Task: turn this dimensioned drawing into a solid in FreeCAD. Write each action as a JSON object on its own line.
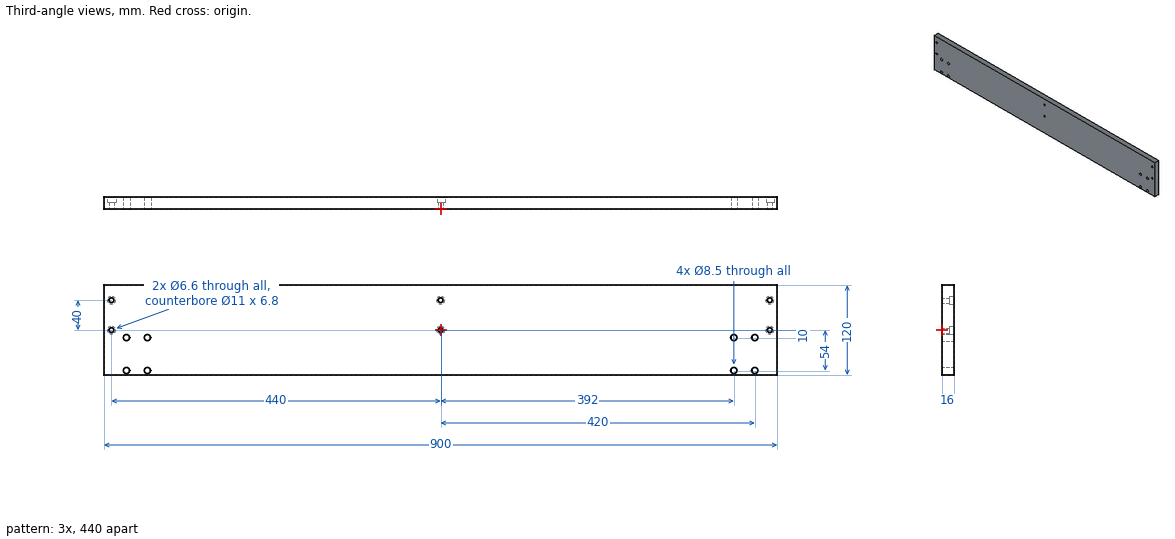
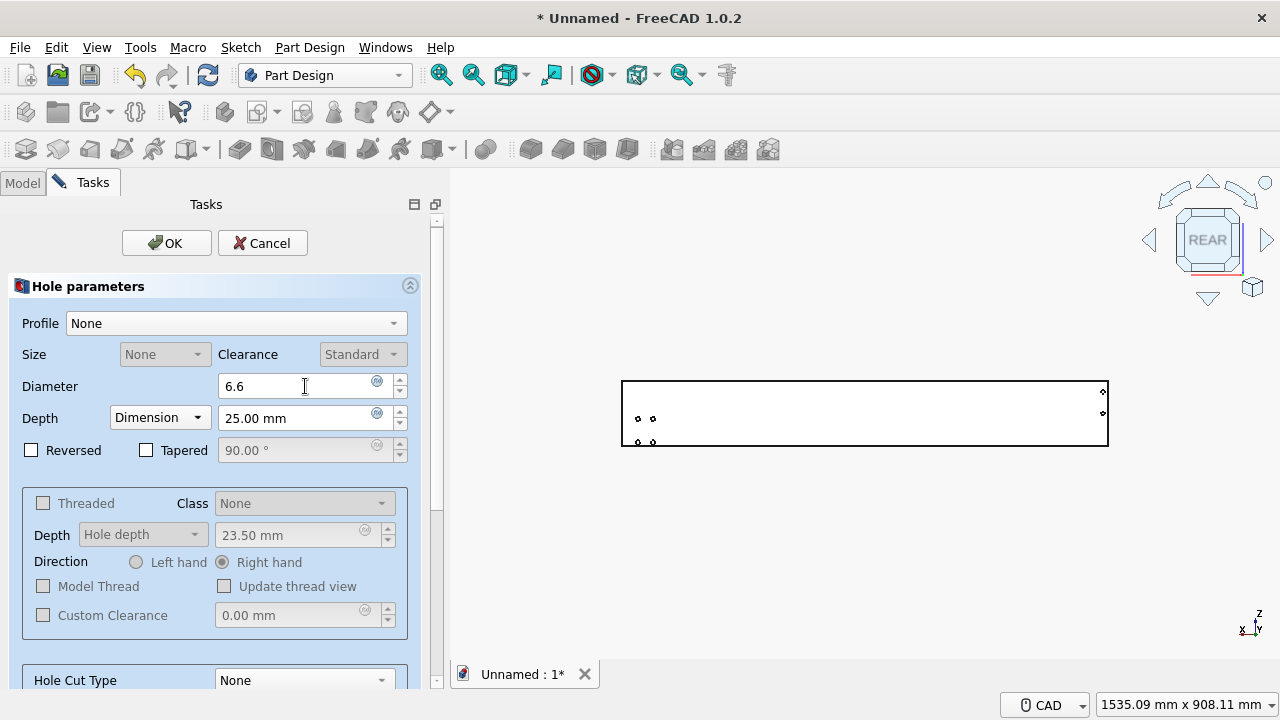
{"action": "left_click", "coordinate": [161, 418]}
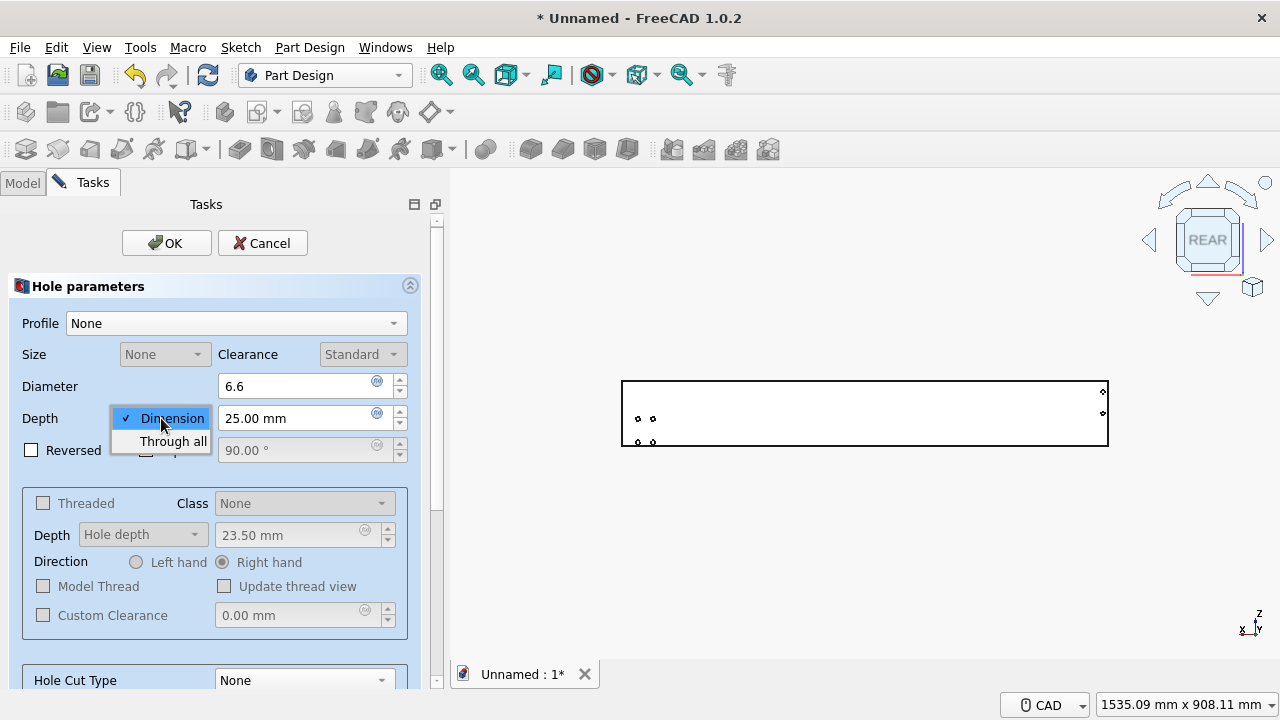
{"action": "left_click", "coordinate": [160, 442]}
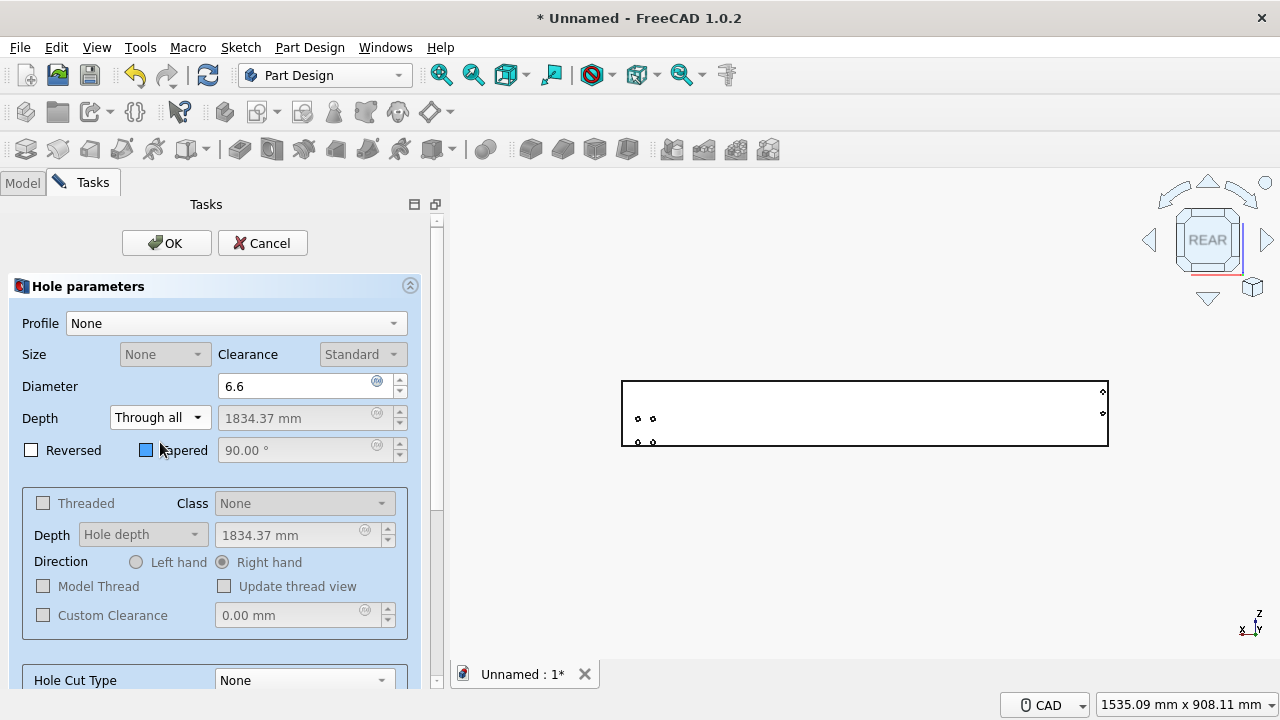
{"action": "scroll", "coordinate": [437, 451], "scroll_direction": "down", "scroll_amount": 2}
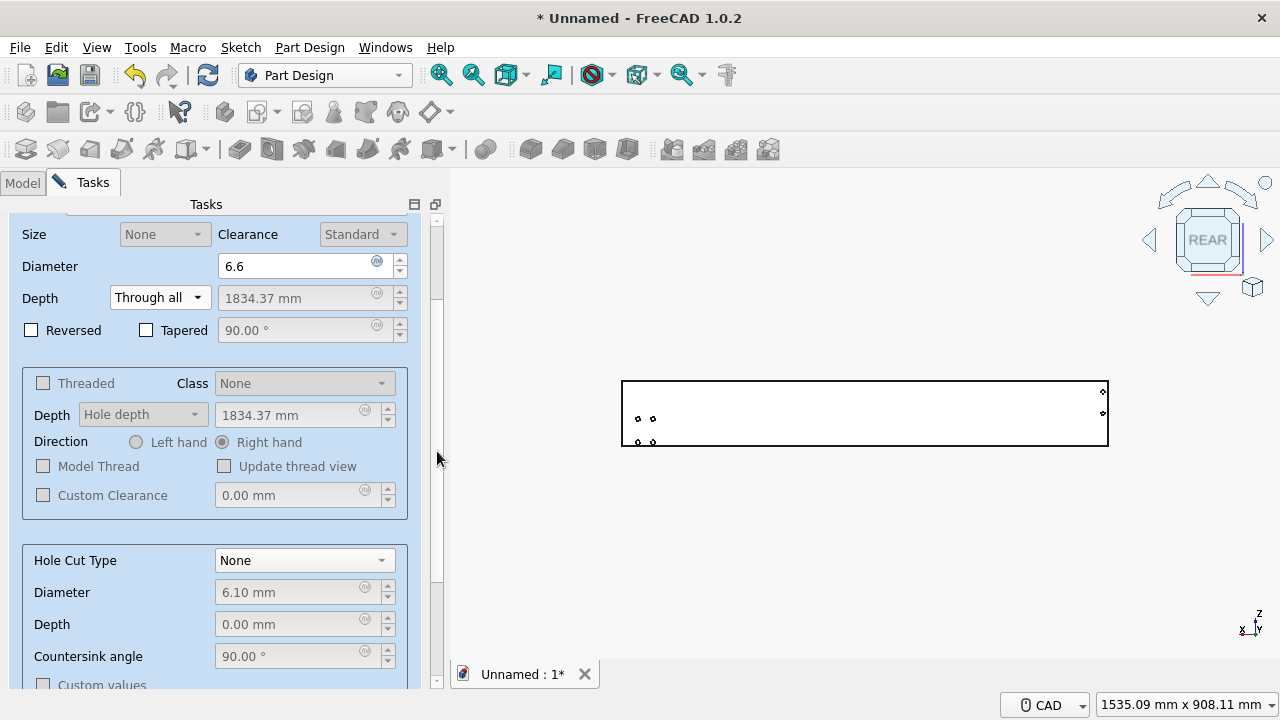
{"action": "left_click", "coordinate": [306, 560]}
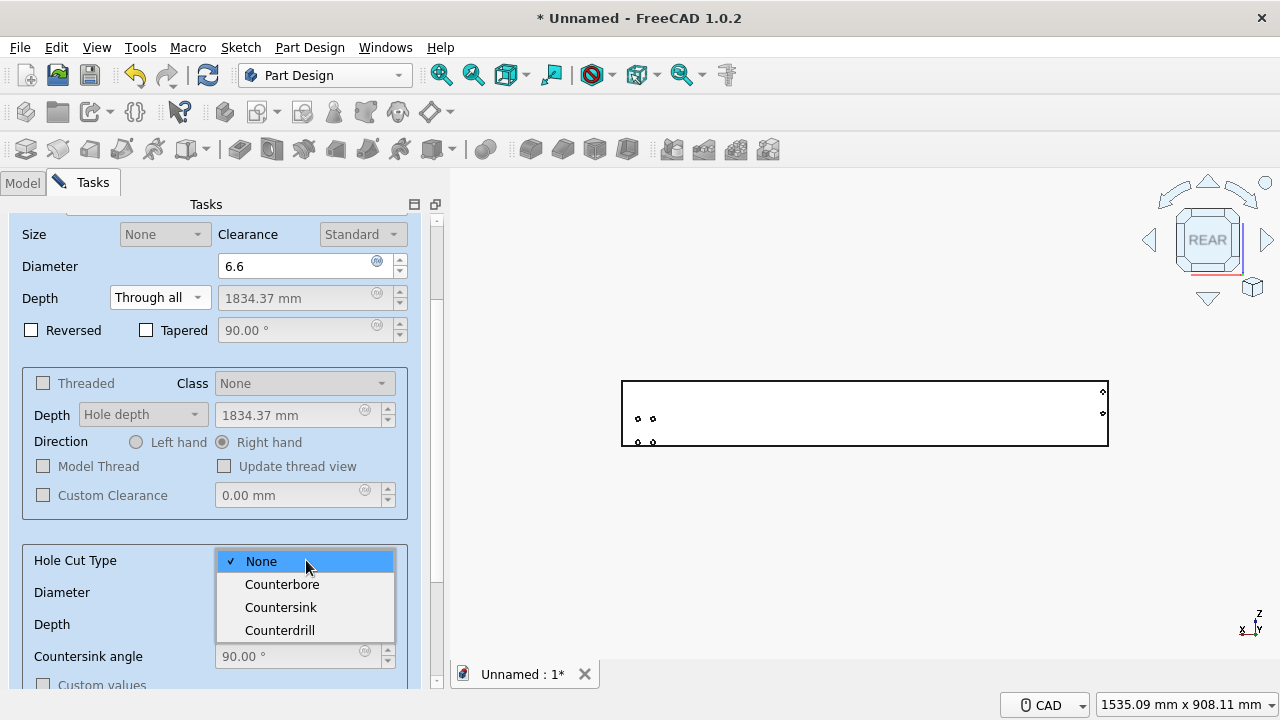
{"action": "left_click", "coordinate": [304, 584]}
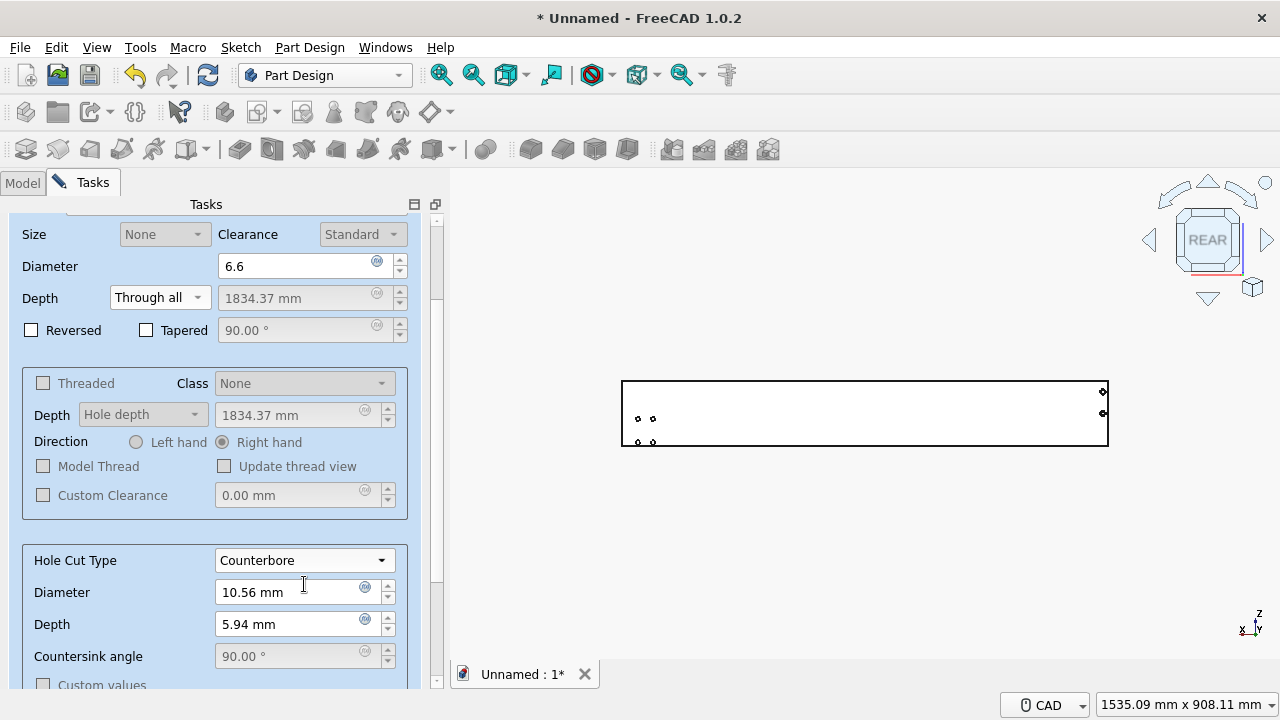
{"action": "triple_click", "coordinate": [298, 592]}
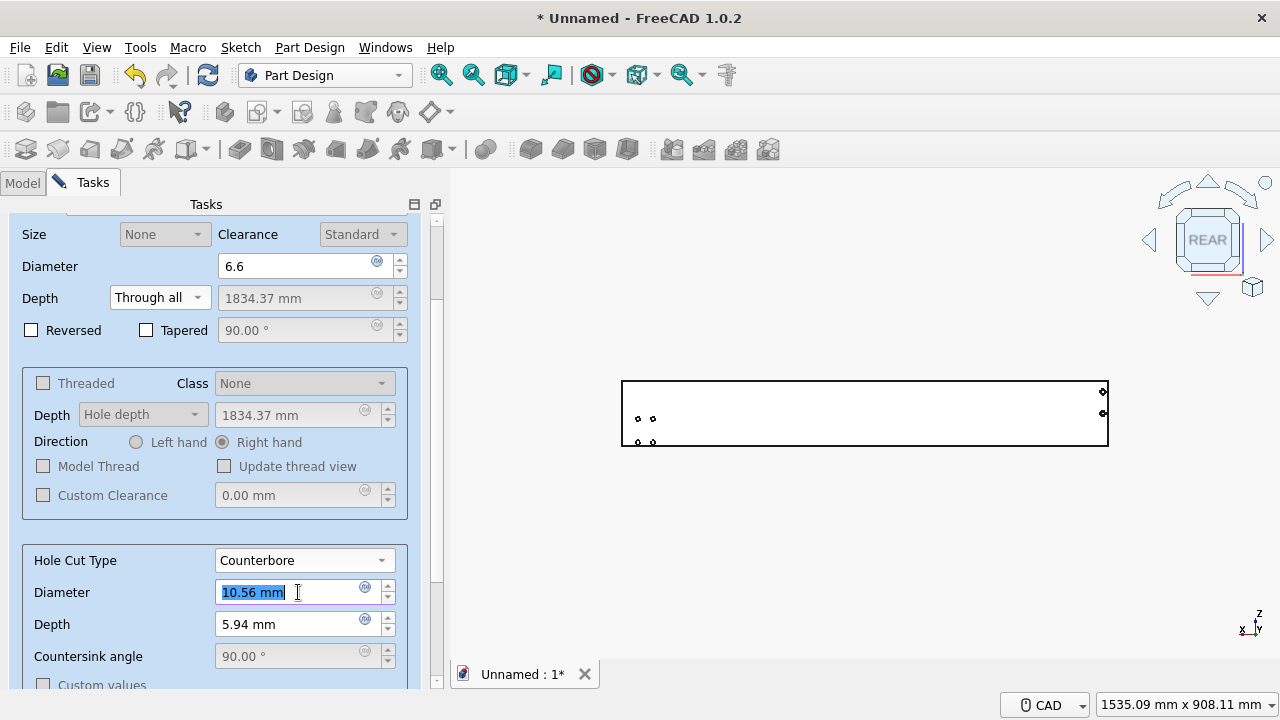
{"action": "type", "text": "11"}
{"action": "key", "text": "Tab"}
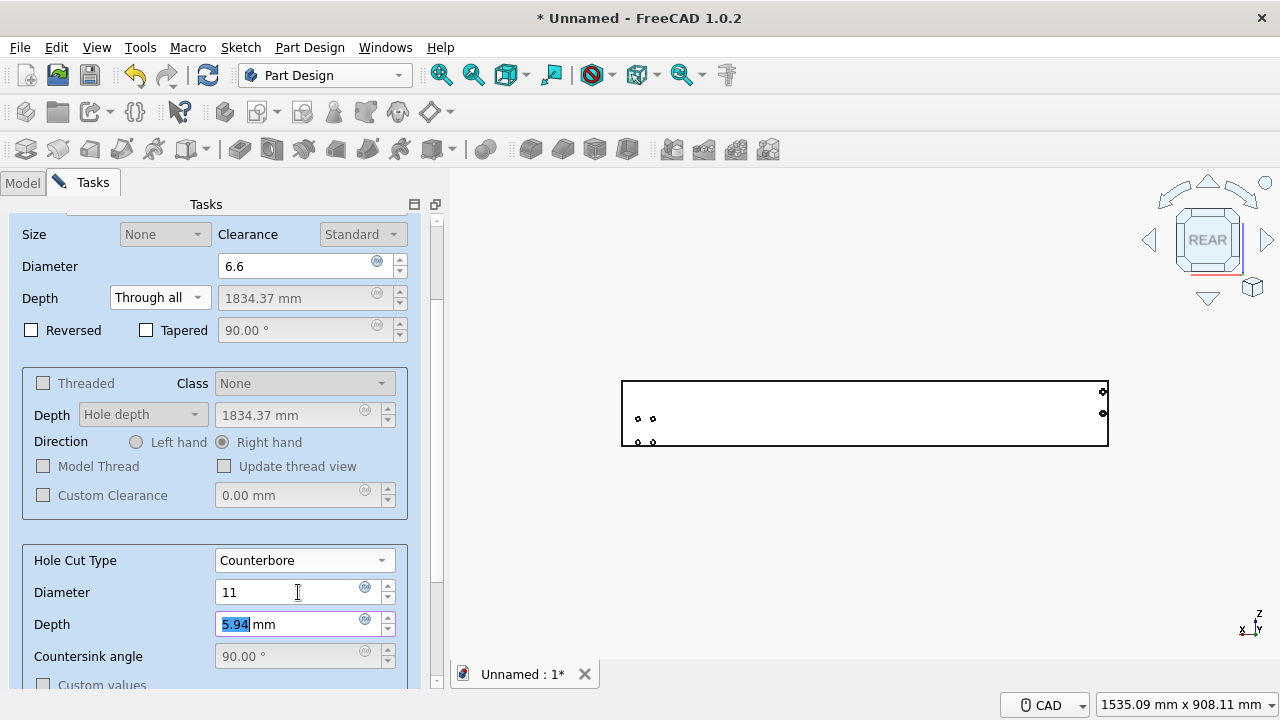
{"action": "type", "text": "6.8"}
{"action": "key", "text": "Tab"}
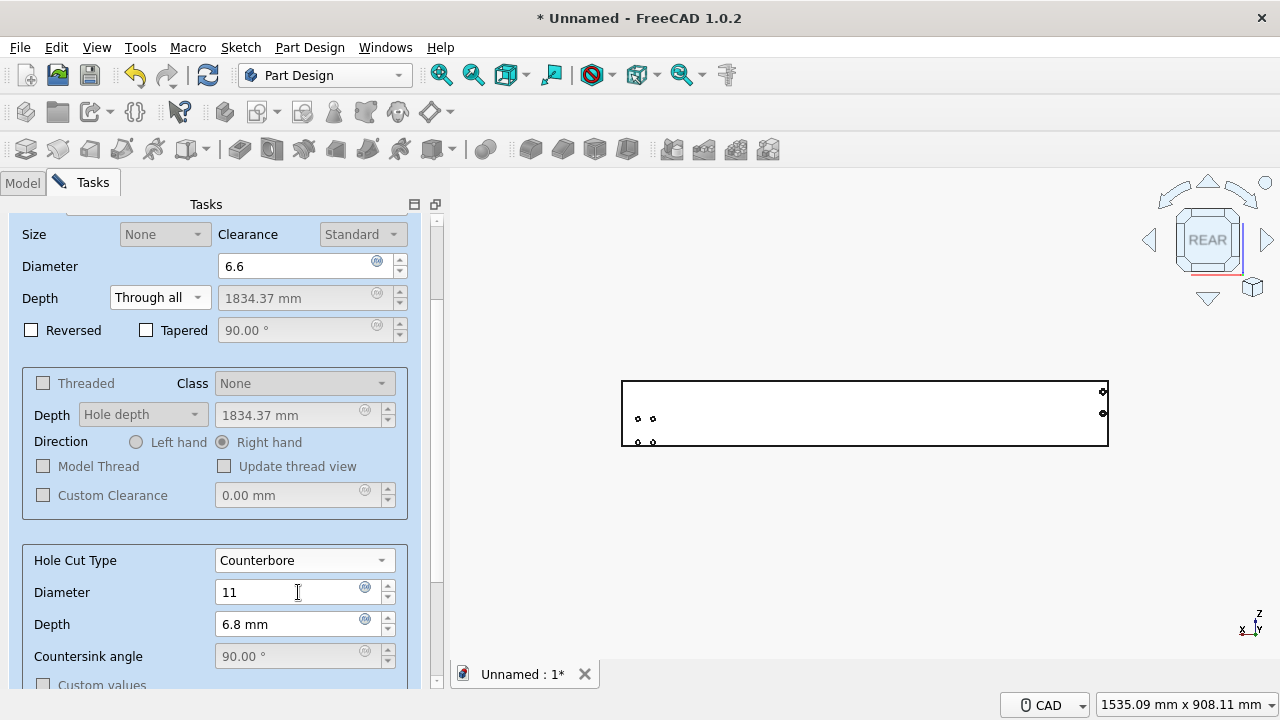
{"action": "scroll", "coordinate": [437, 451], "scroll_direction": "up", "scroll_amount": 3}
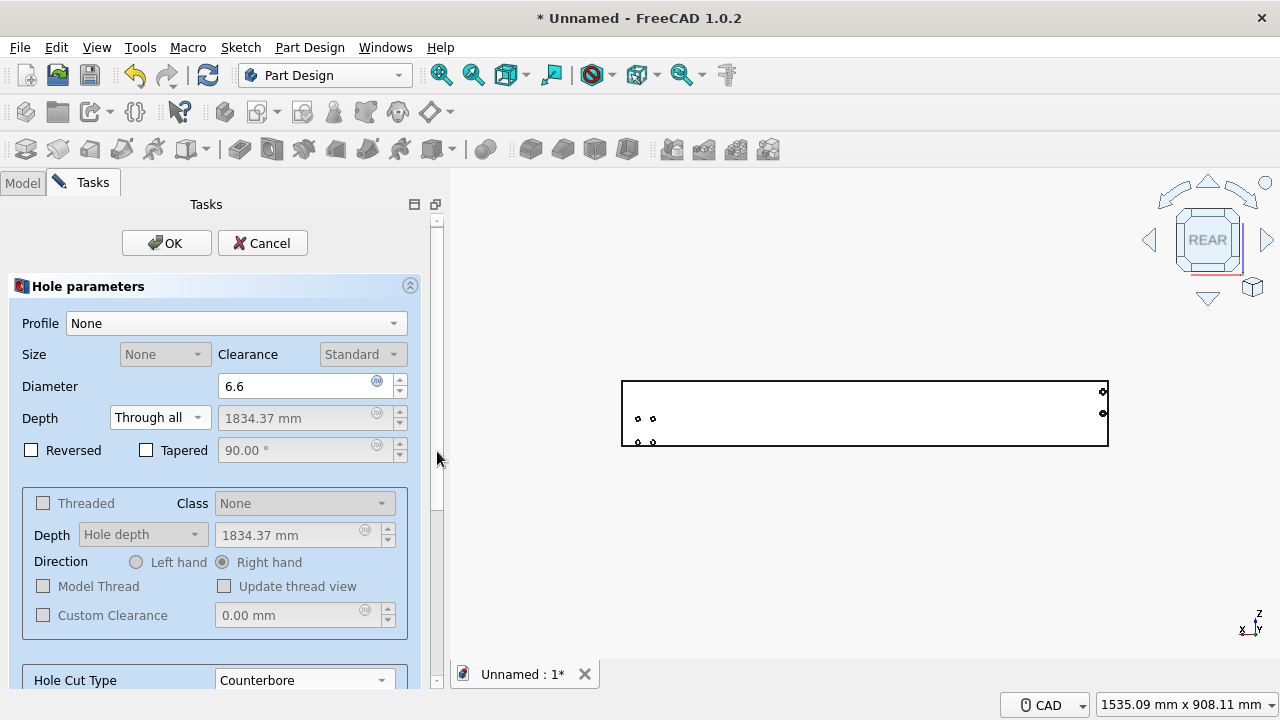
{"action": "left_click", "coordinate": [167, 243]}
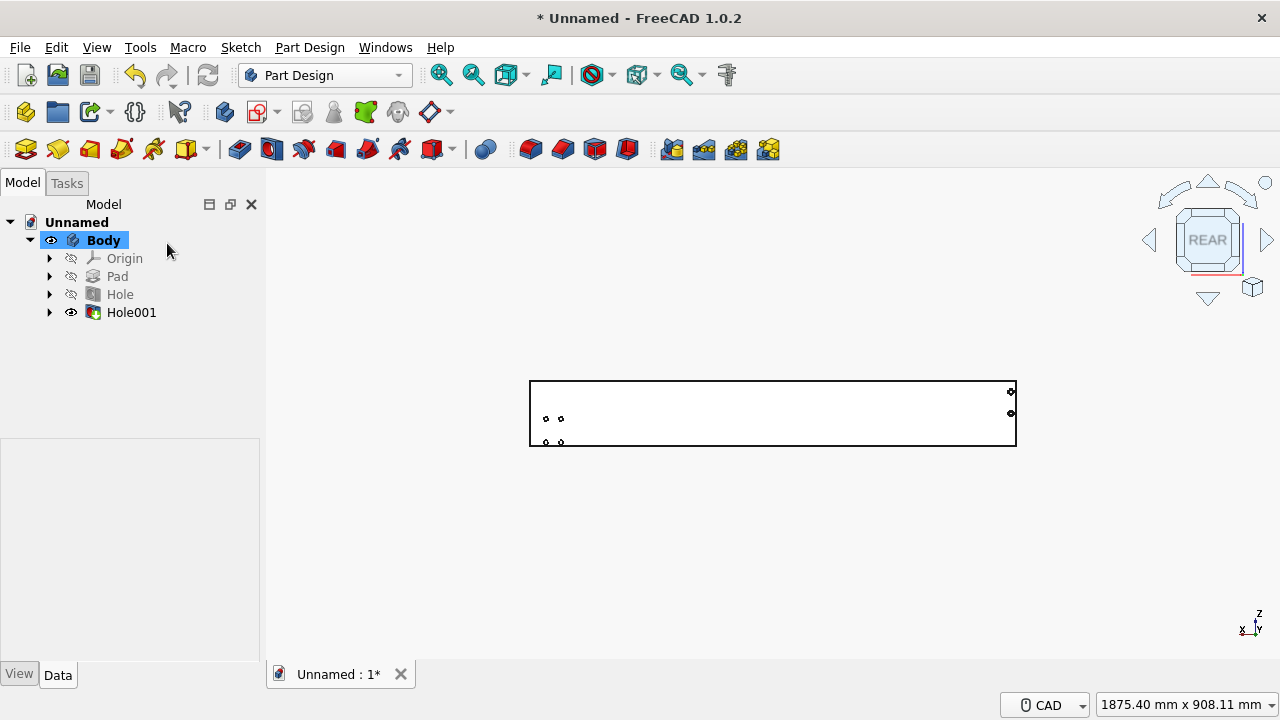
{"action": "left_click", "coordinate": [116, 312]}